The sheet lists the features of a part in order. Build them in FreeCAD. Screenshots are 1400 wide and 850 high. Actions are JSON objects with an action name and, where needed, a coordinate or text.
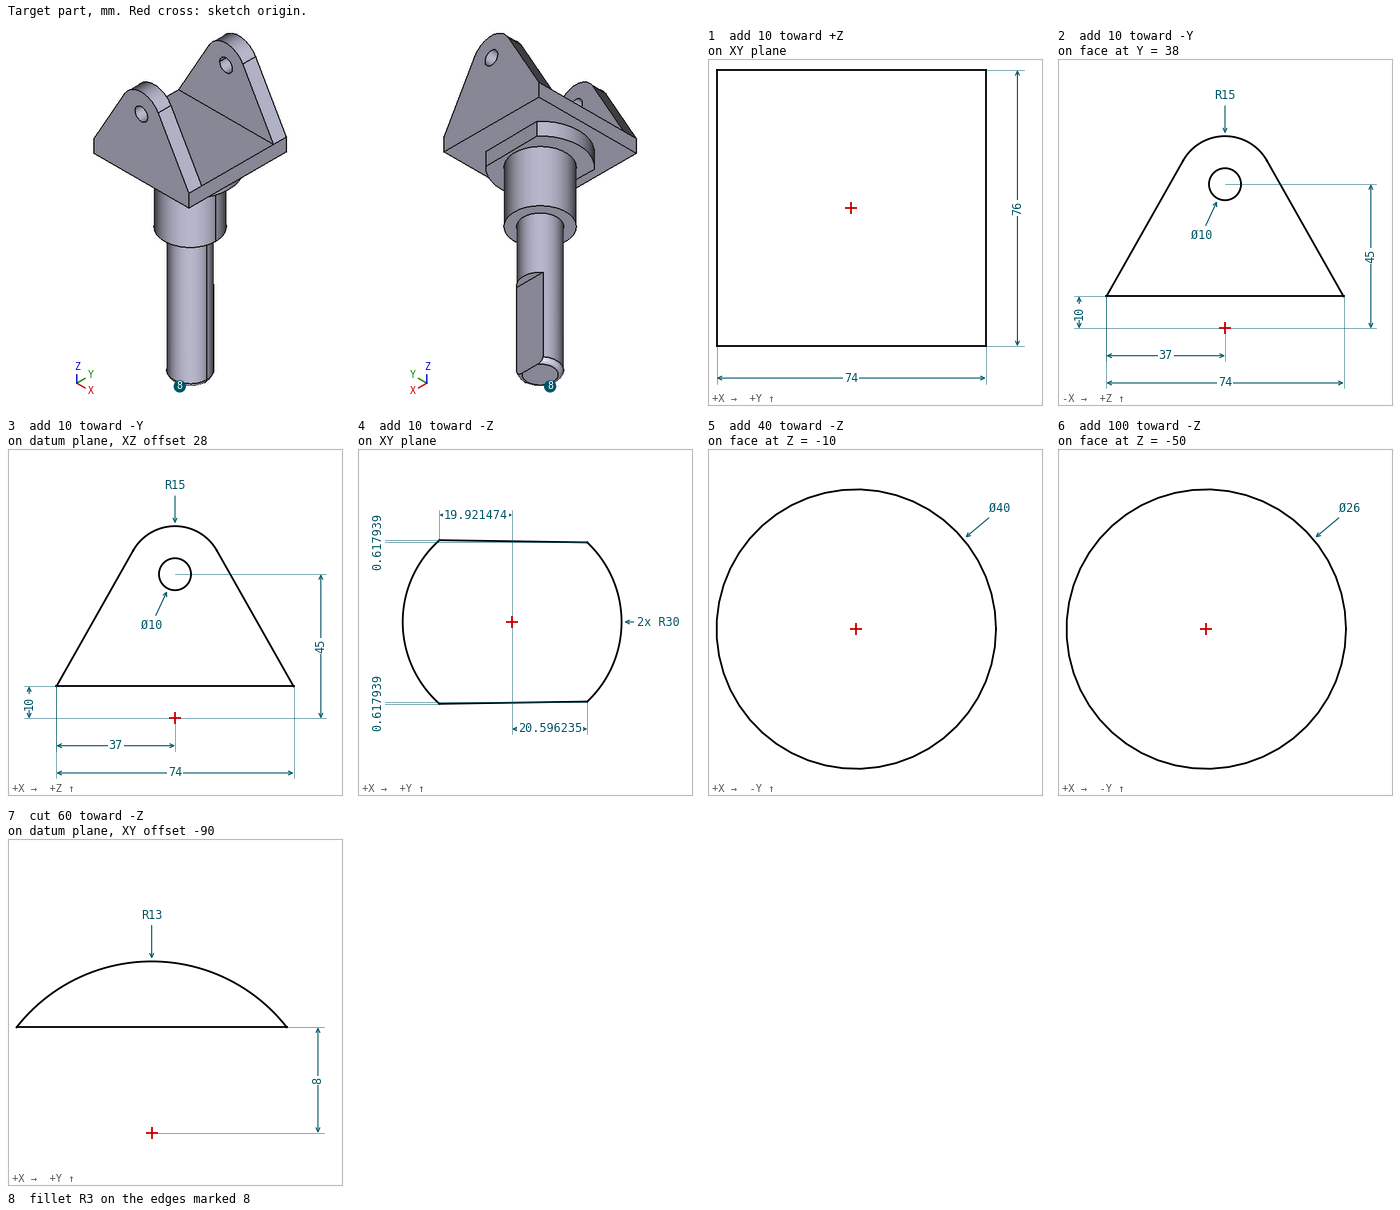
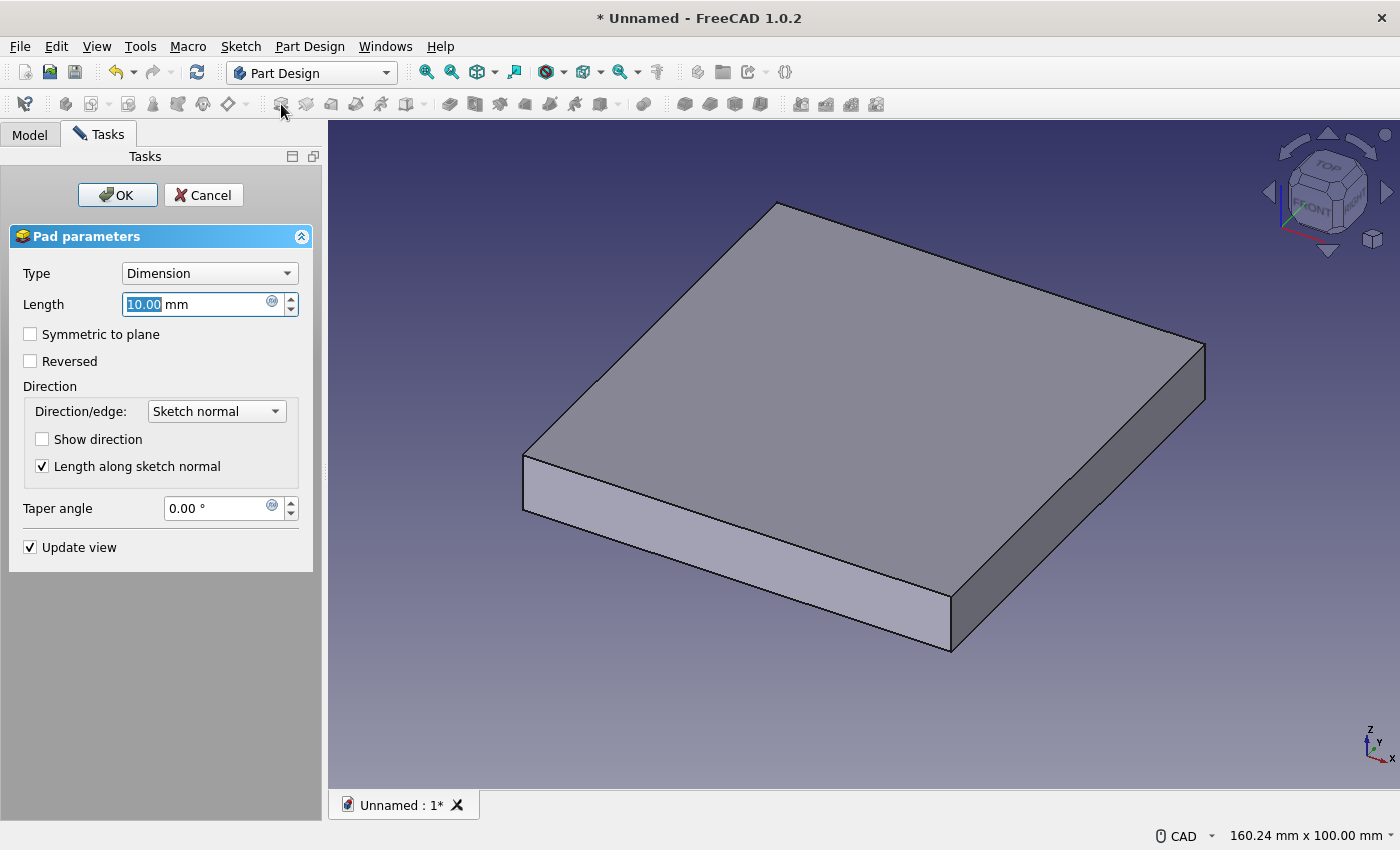
{"action": "type", "text": "10"}
{"action": "key", "text": "Tab"}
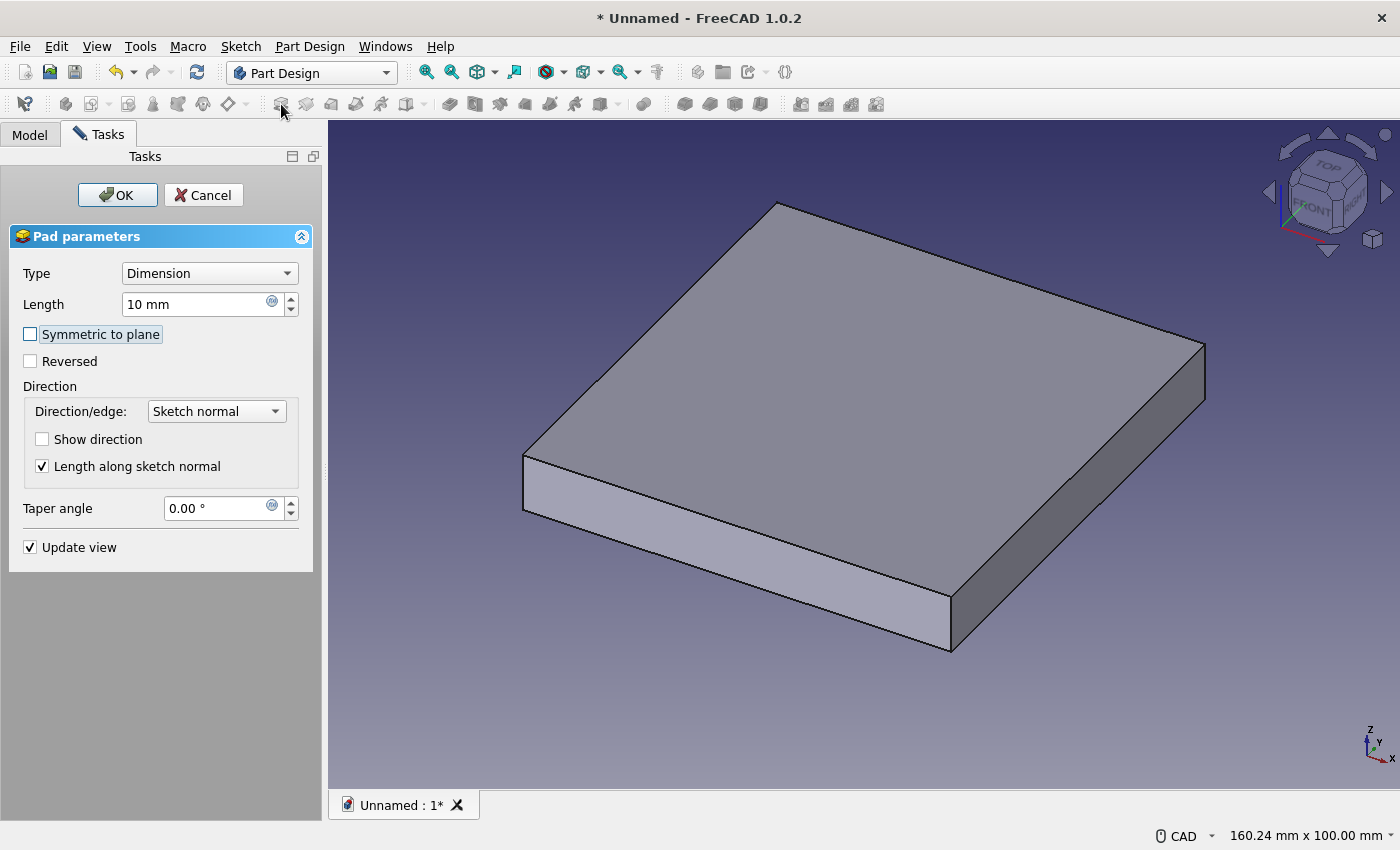
{"action": "left_click", "coordinate": [118, 195]}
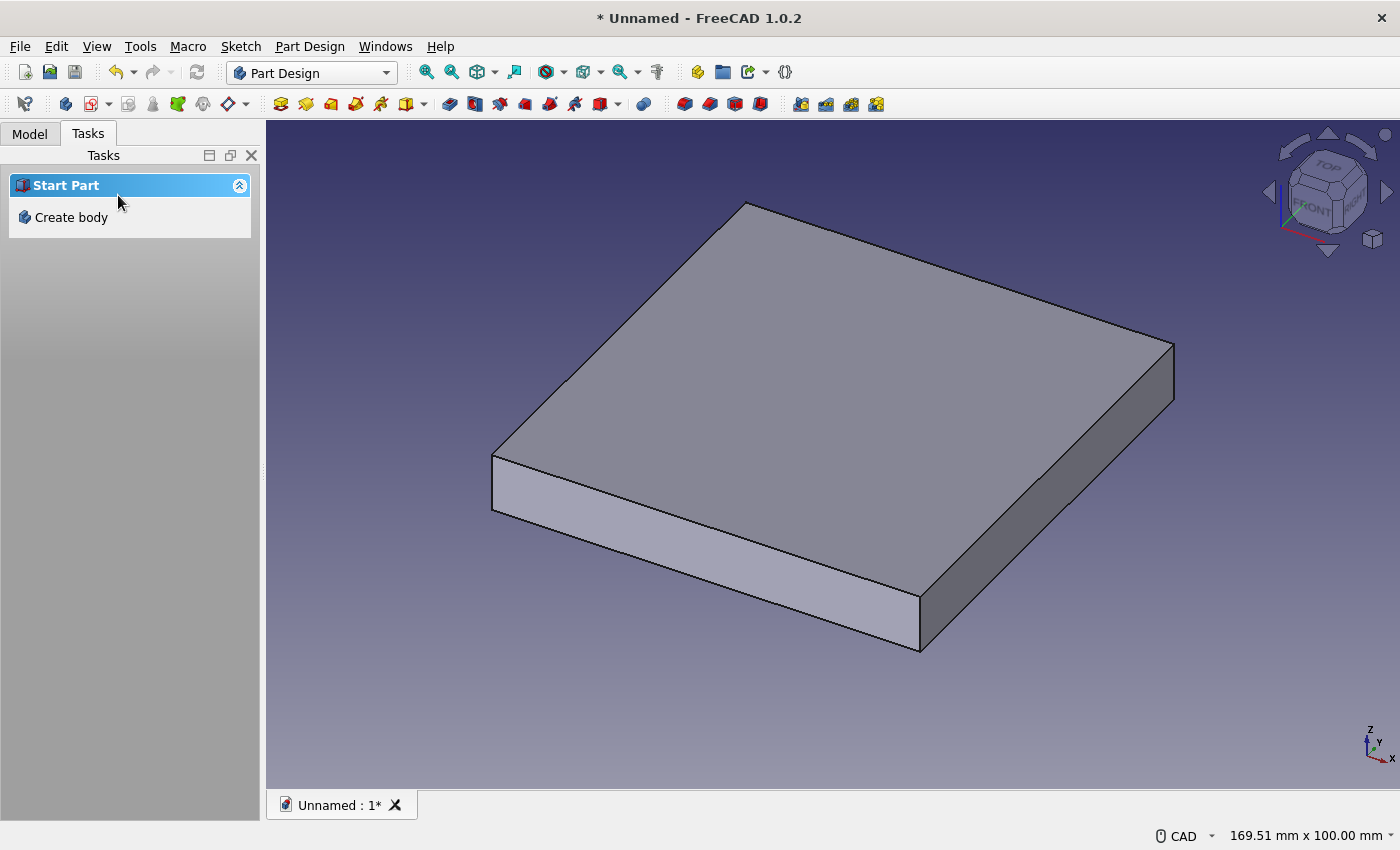
{"action": "key", "text": "4"}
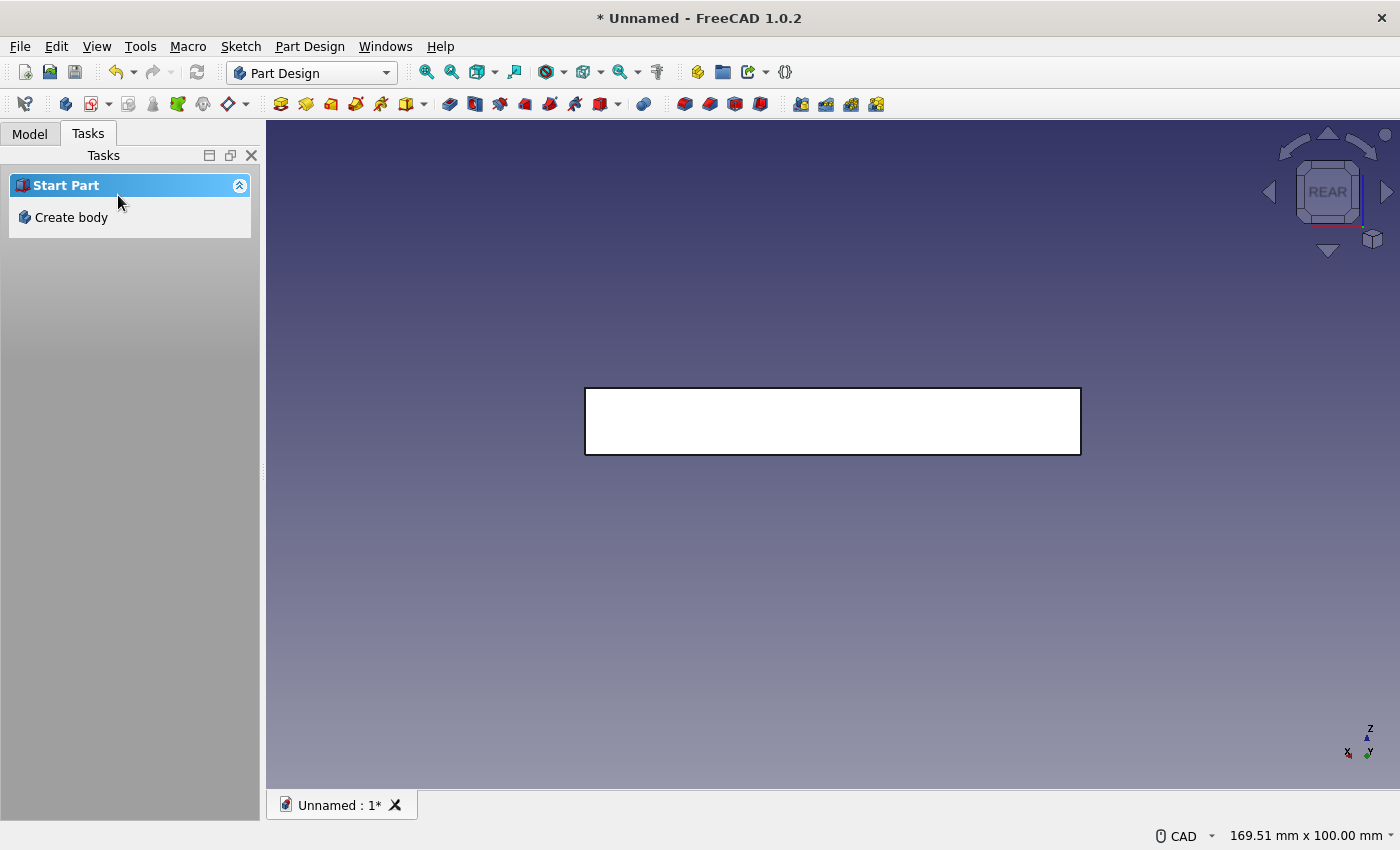
{"action": "left_click", "coordinate": [427, 72]}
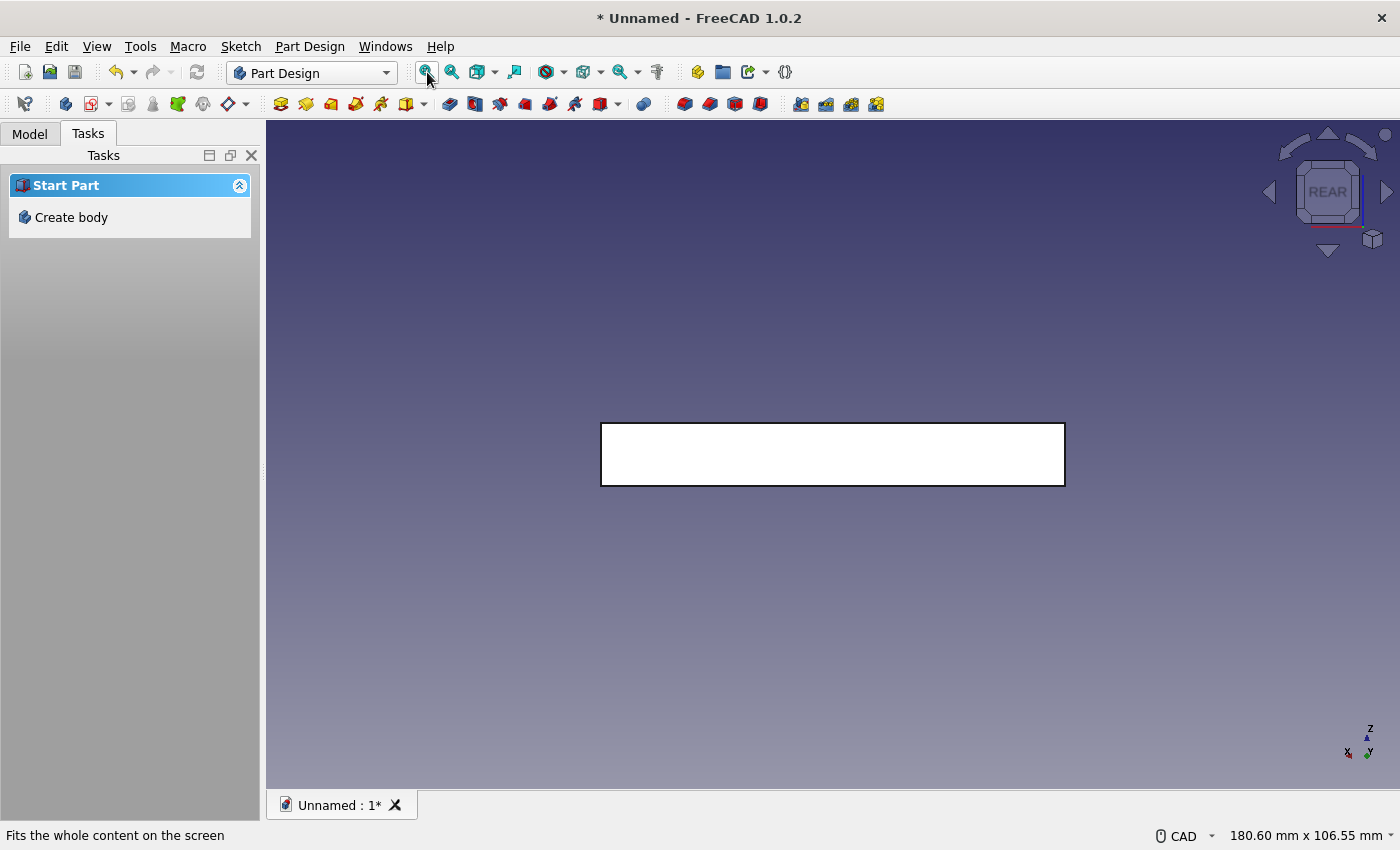
{"action": "left_click", "coordinate": [634, 454]}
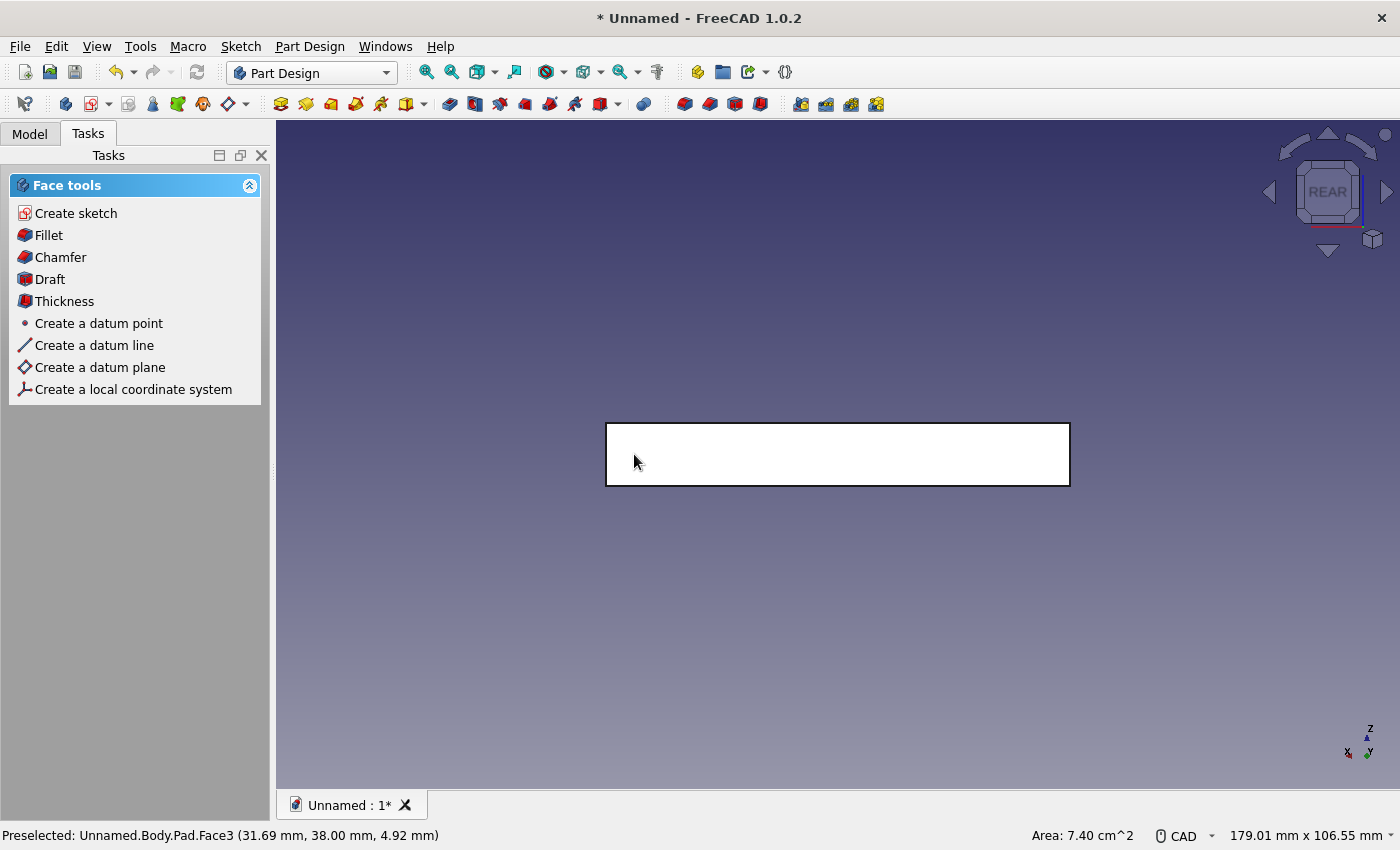
{"action": "left_click", "coordinate": [90, 104]}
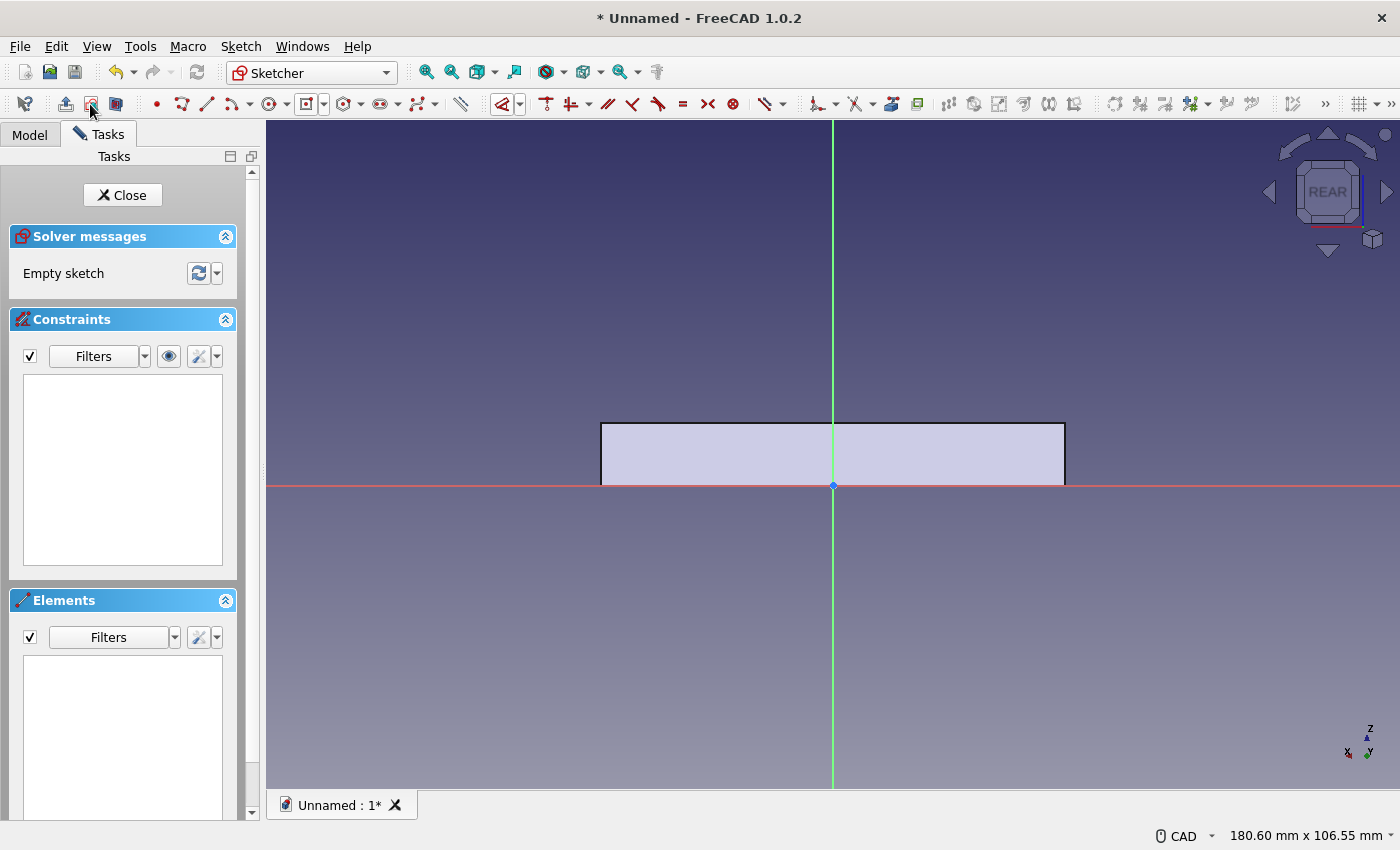
{"action": "scroll", "coordinate": [455, 761], "scroll_direction": "down", "scroll_amount": 1}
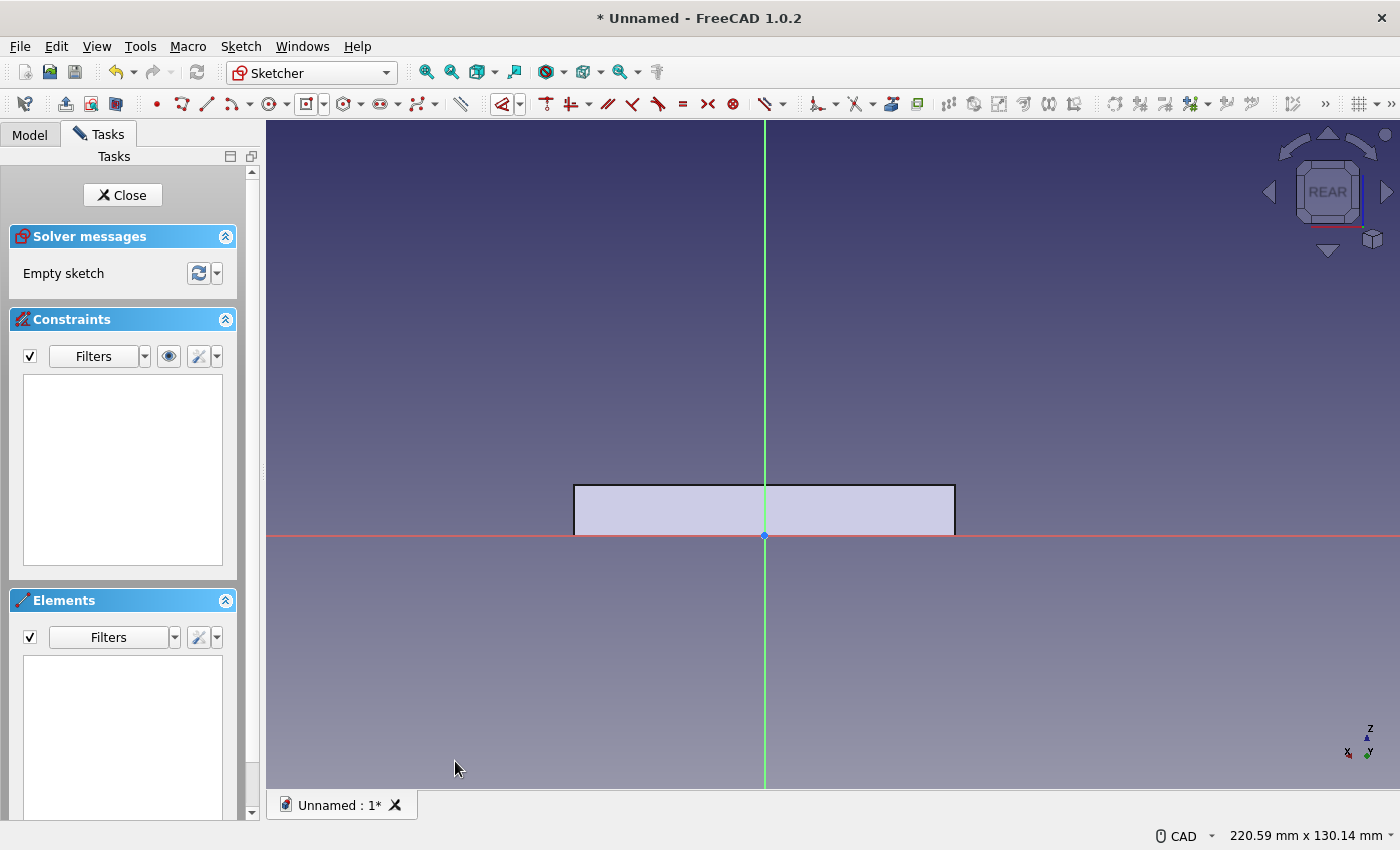
{"action": "scroll", "coordinate": [765, 234], "scroll_direction": "up", "scroll_amount": 2}